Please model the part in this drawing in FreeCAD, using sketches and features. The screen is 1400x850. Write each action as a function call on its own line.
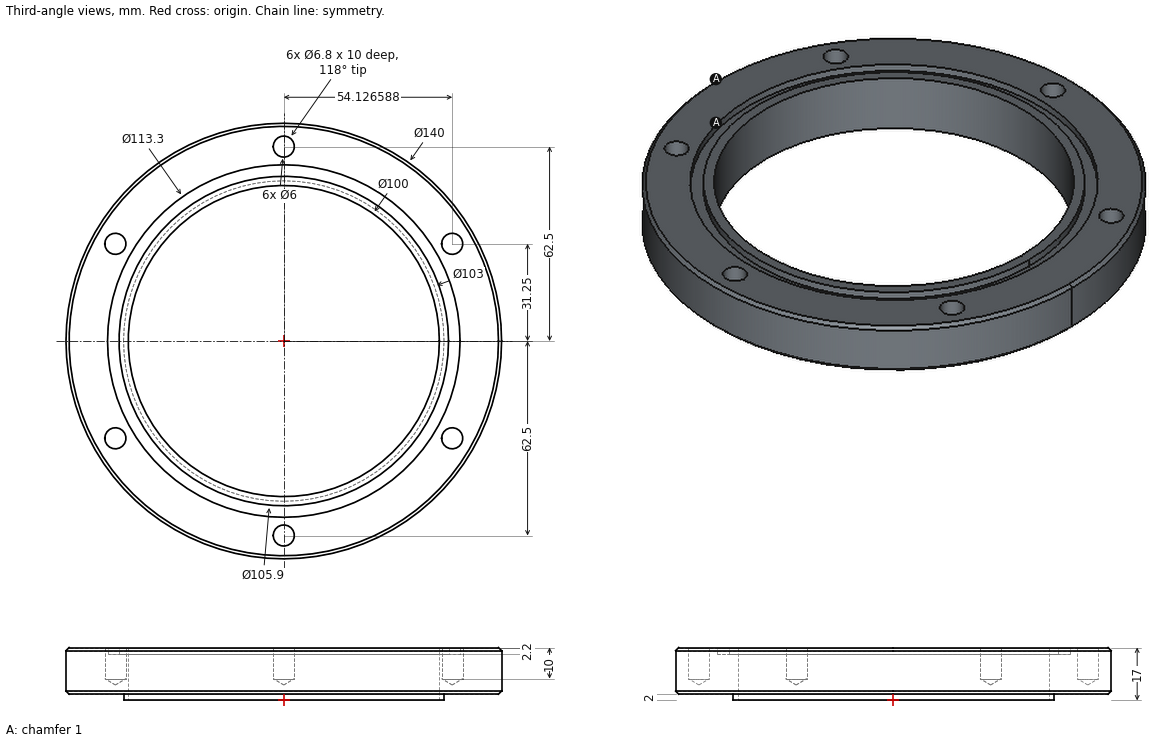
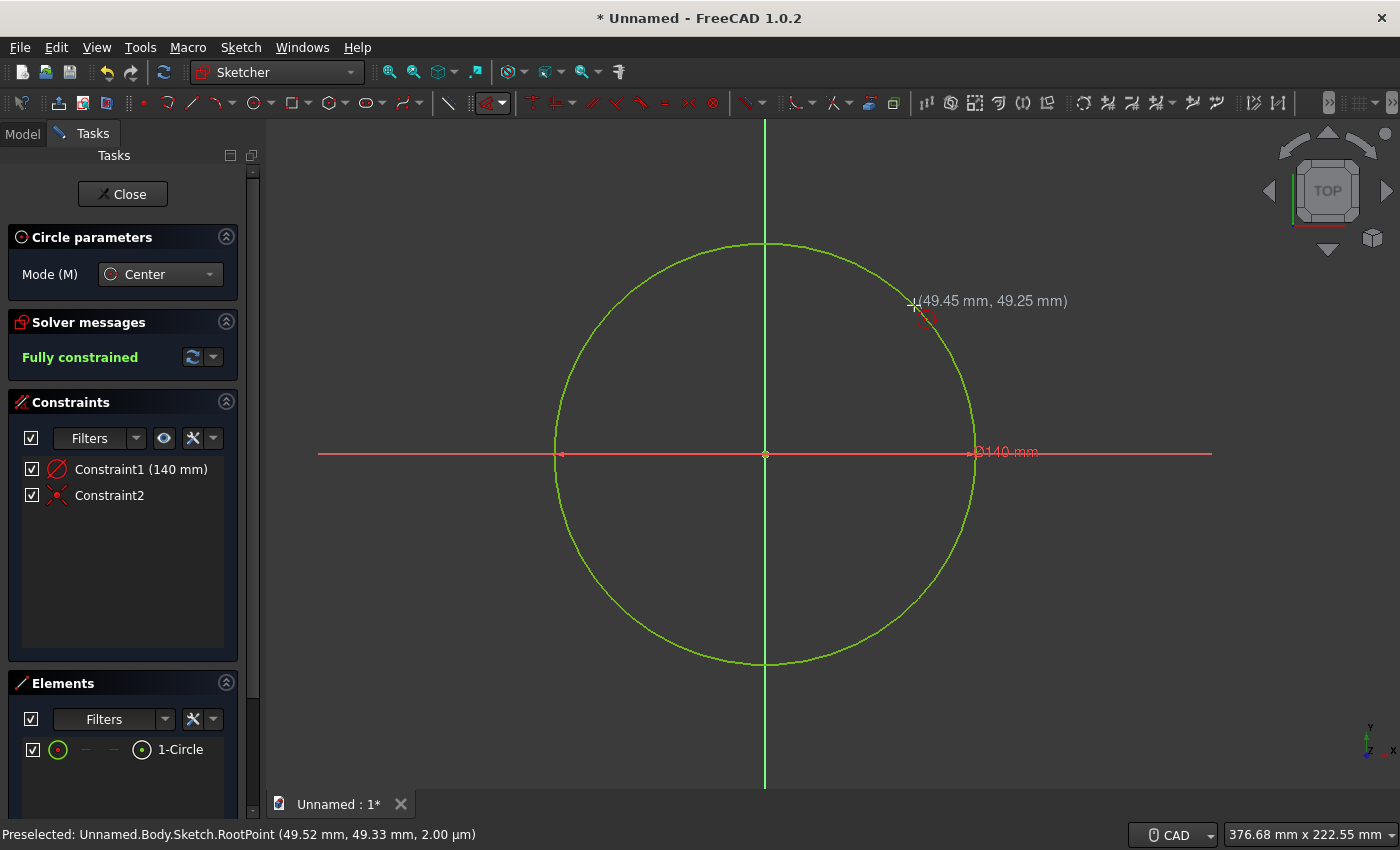
click(765, 454)
move(872, 348)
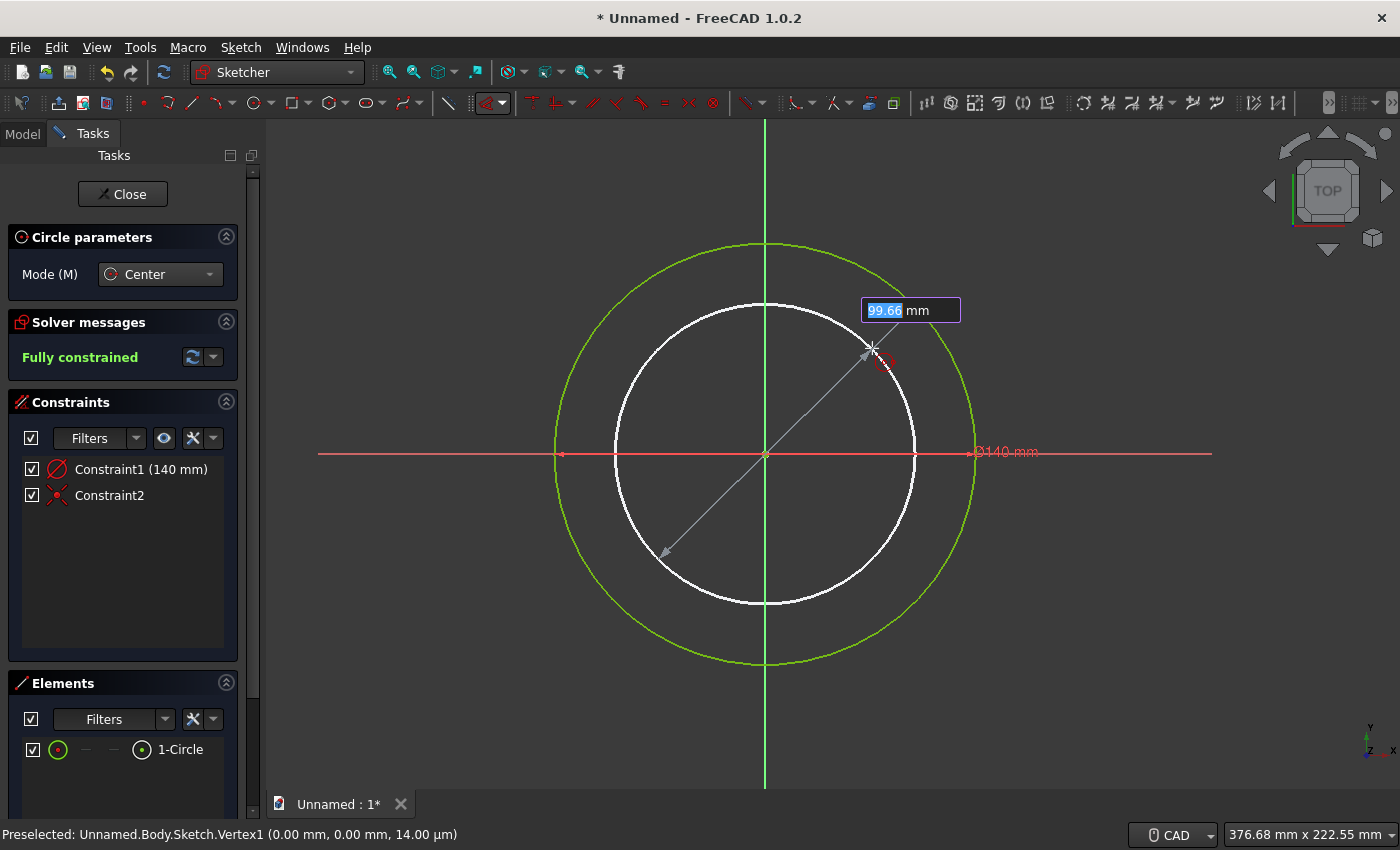
text(100)
key(Return)
key(Escape)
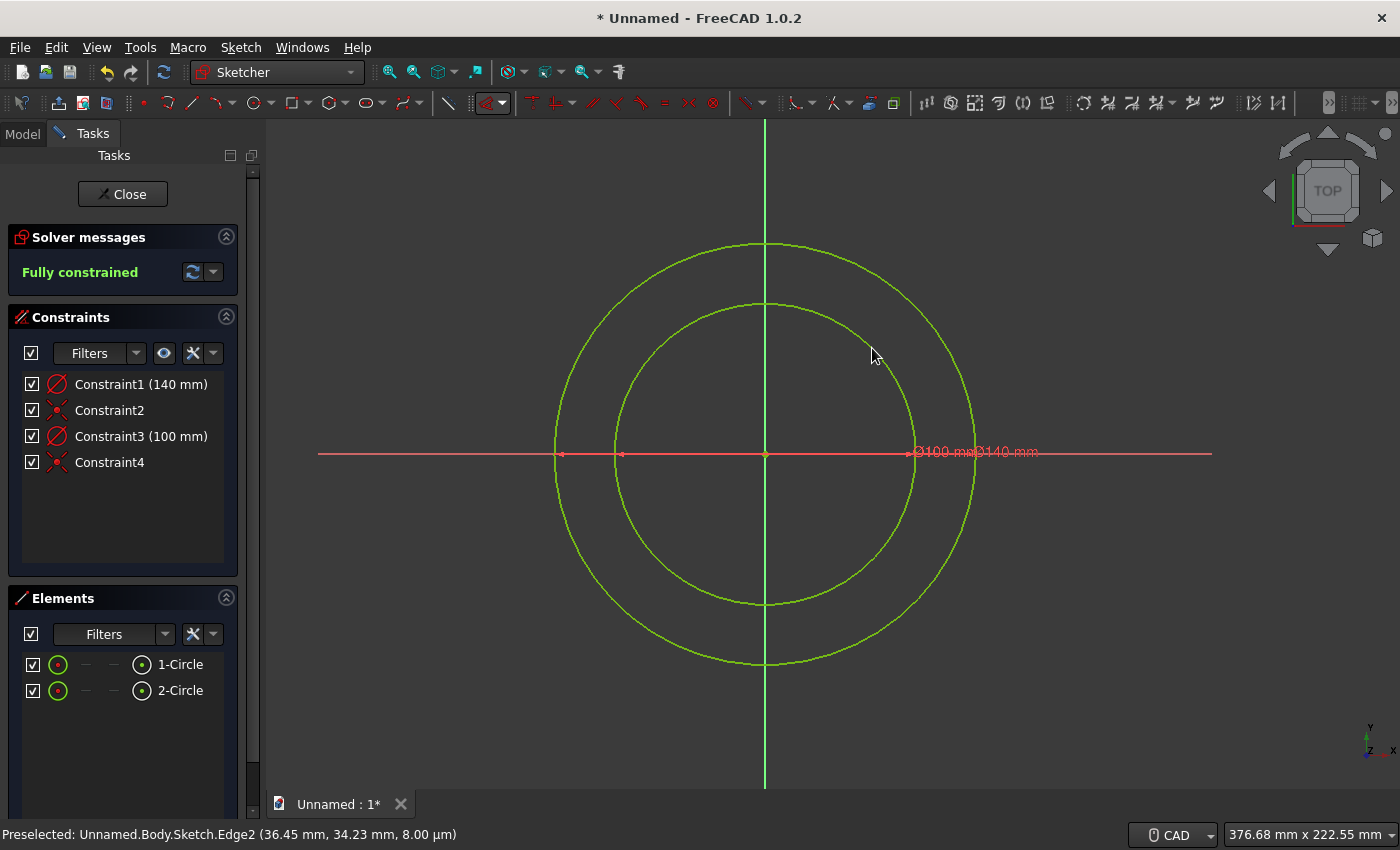
click(123, 194)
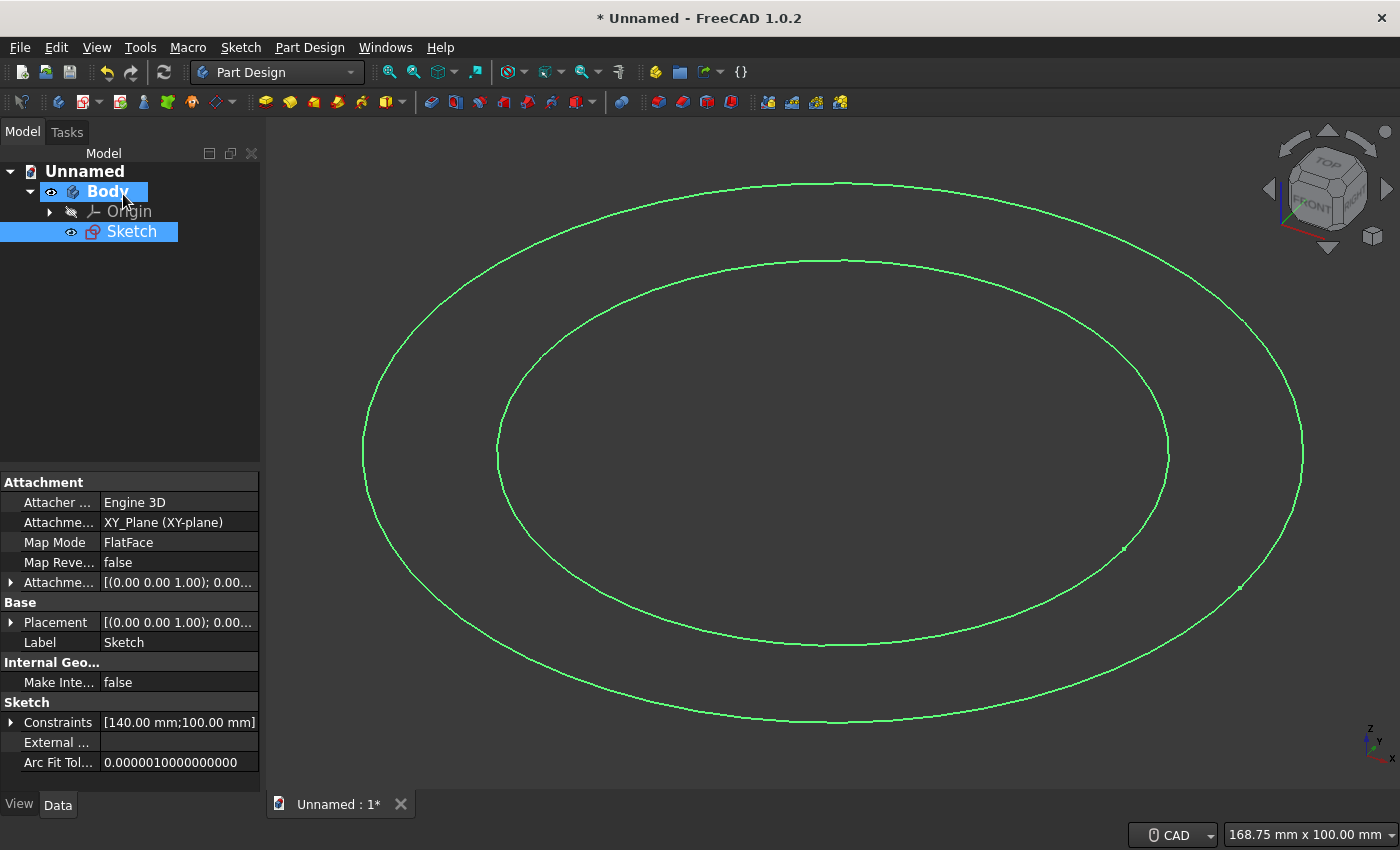
click(266, 102)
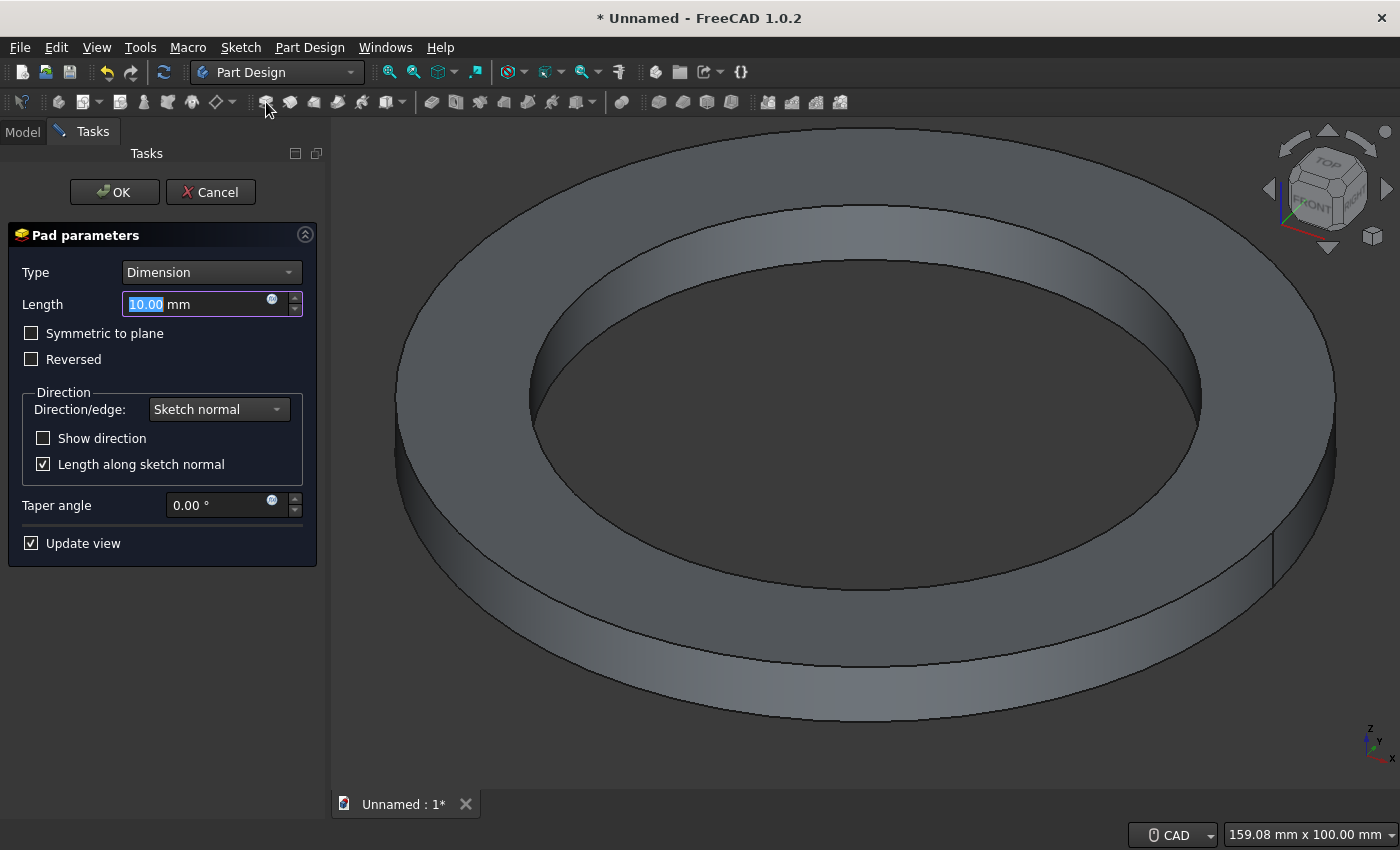
text(17)
key(Tab)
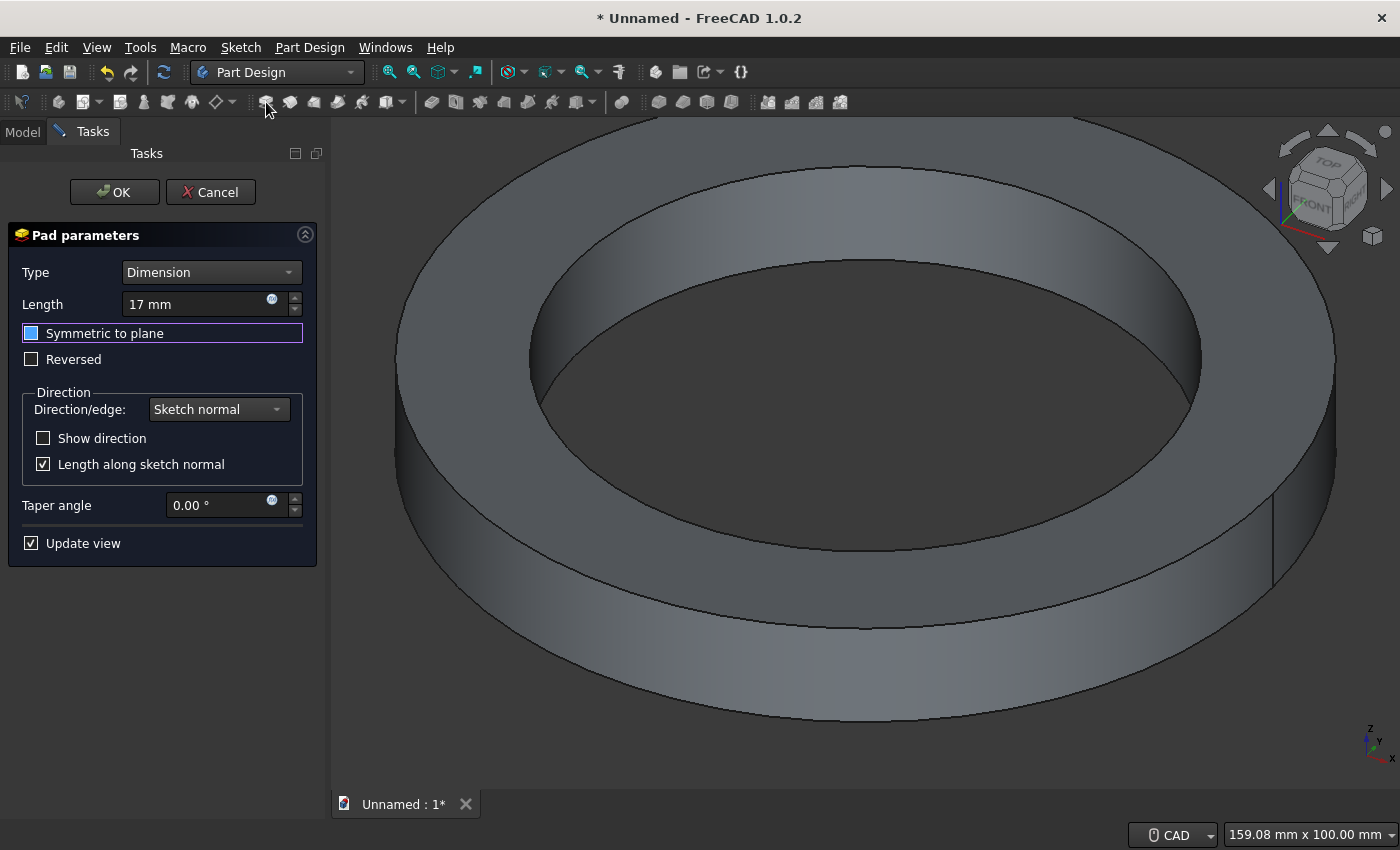
click(115, 192)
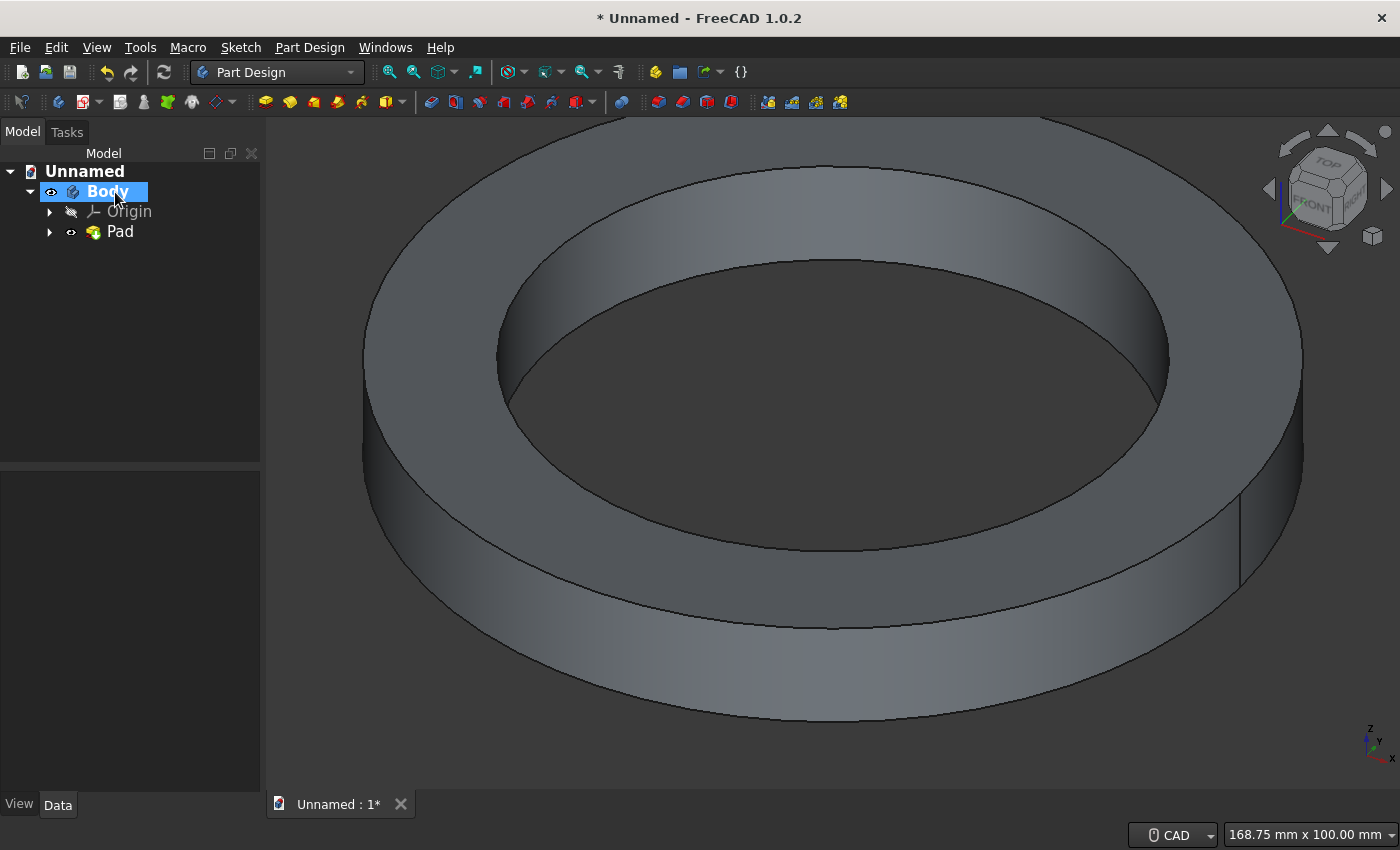
click(390, 72)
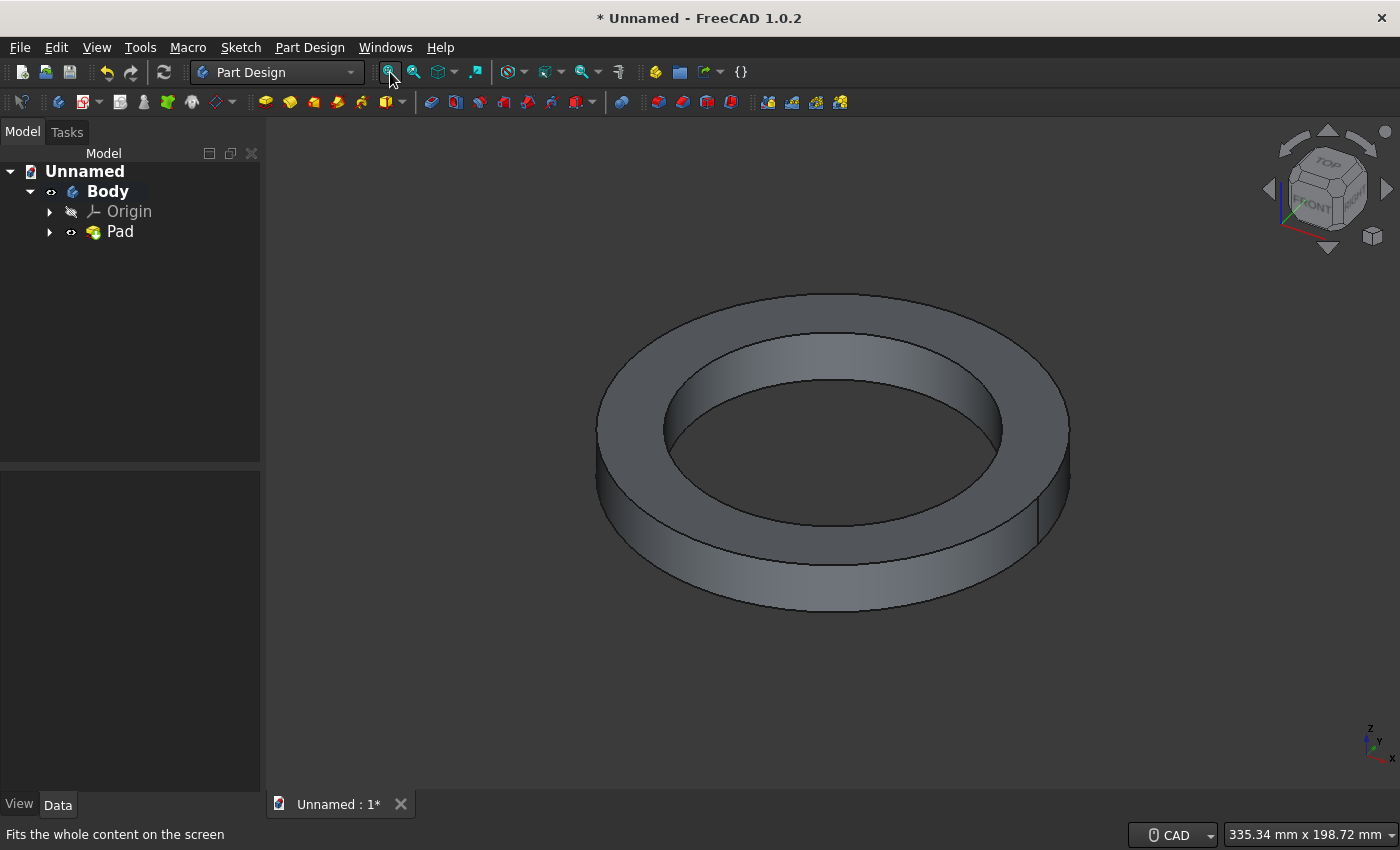
click(1009, 487)